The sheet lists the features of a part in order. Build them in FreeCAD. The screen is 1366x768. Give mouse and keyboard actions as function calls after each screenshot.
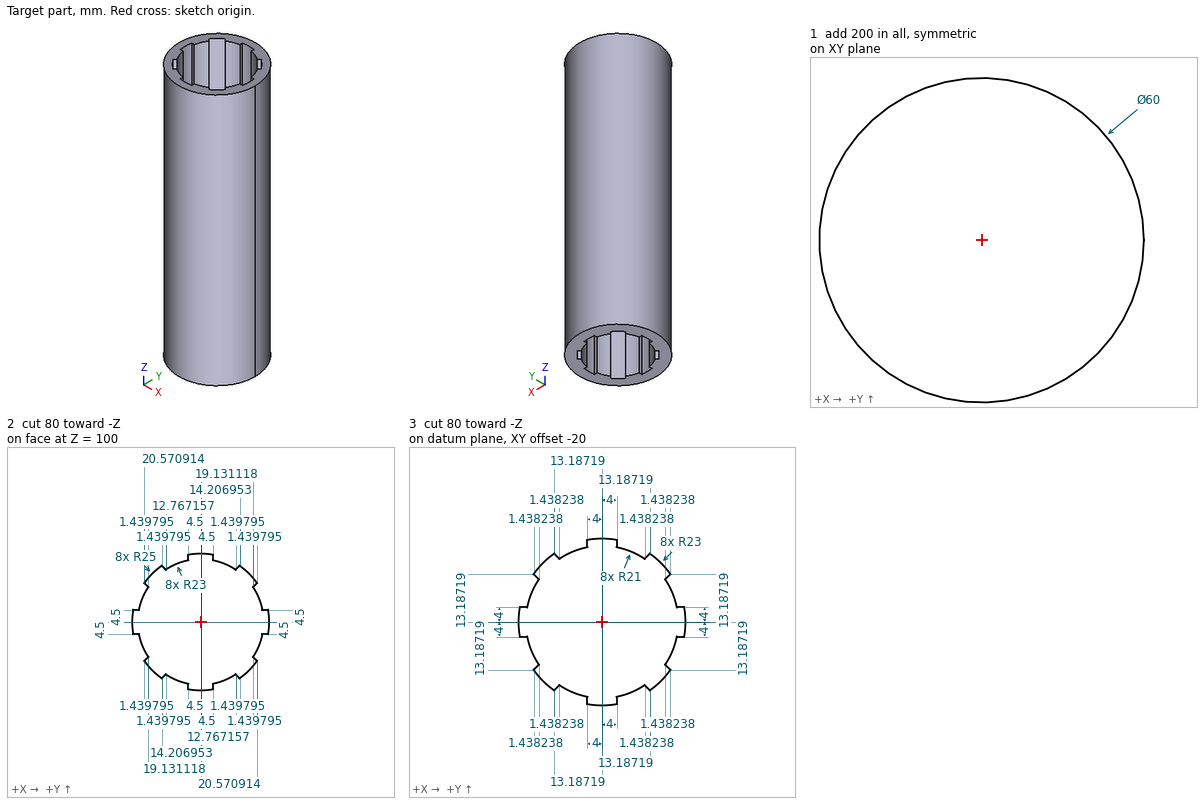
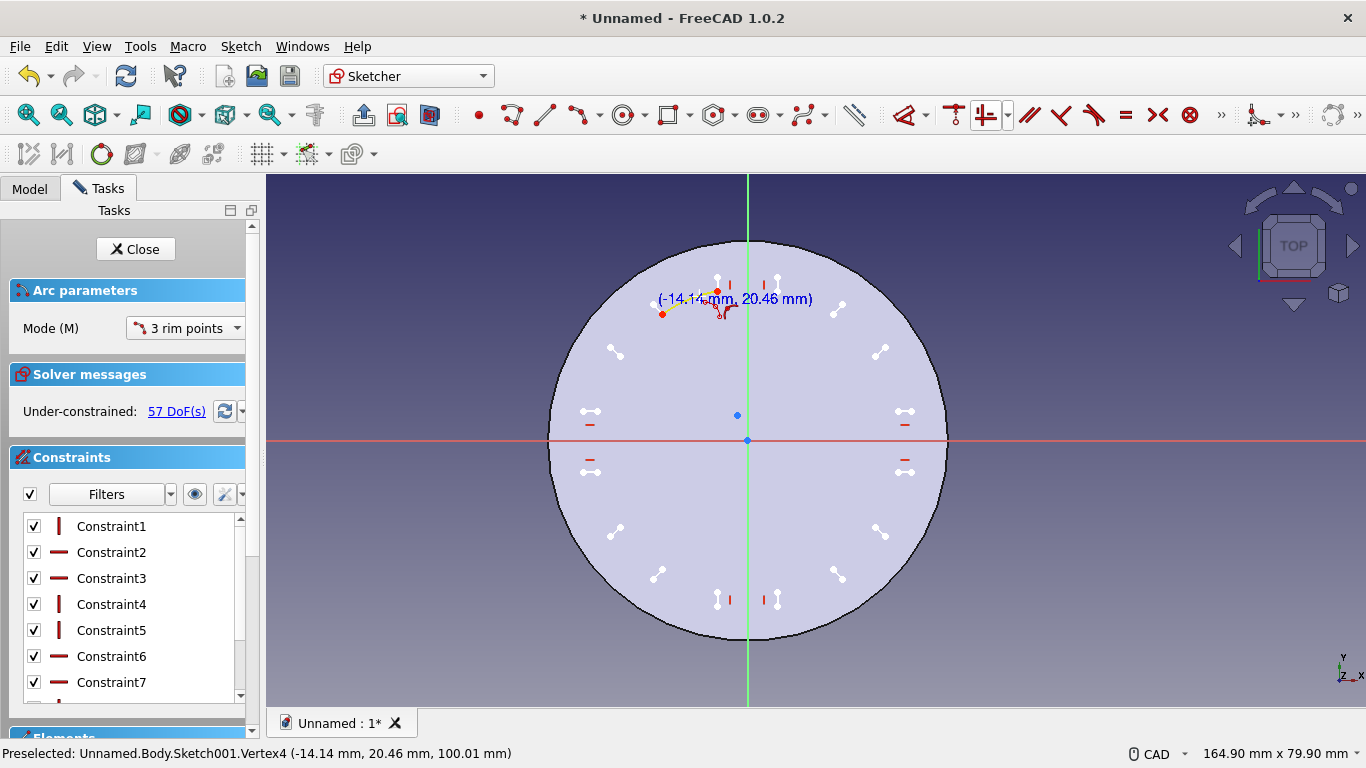
scroll(611, 346, up, 5)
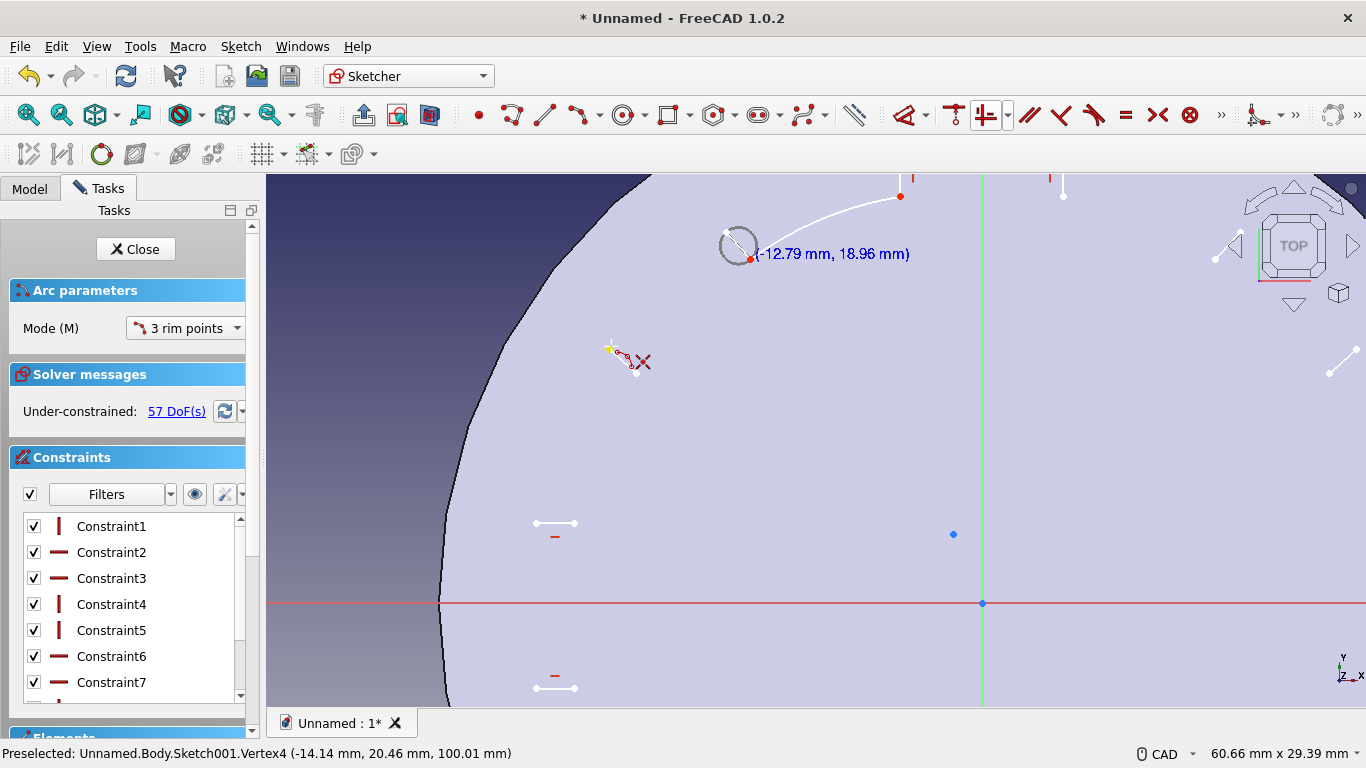
click(609, 349)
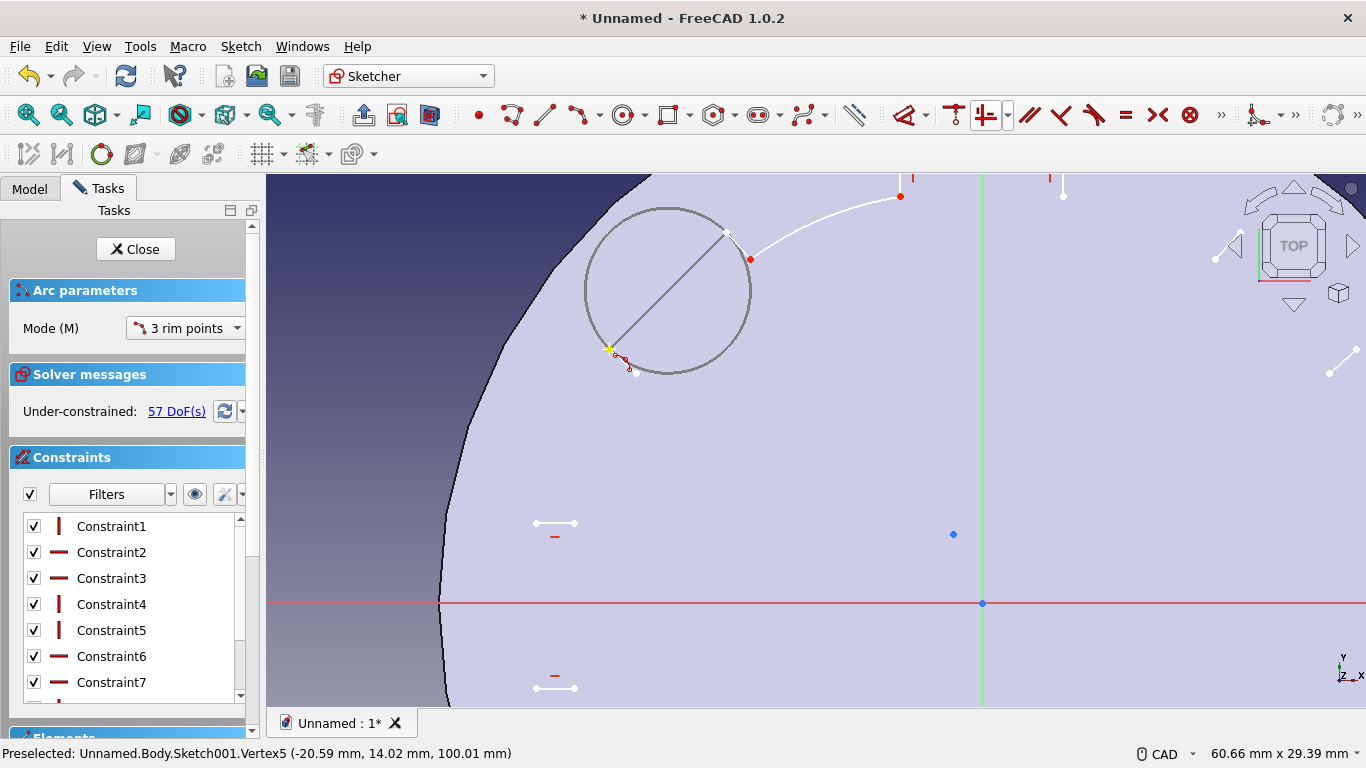
scroll(662, 283, up, 4)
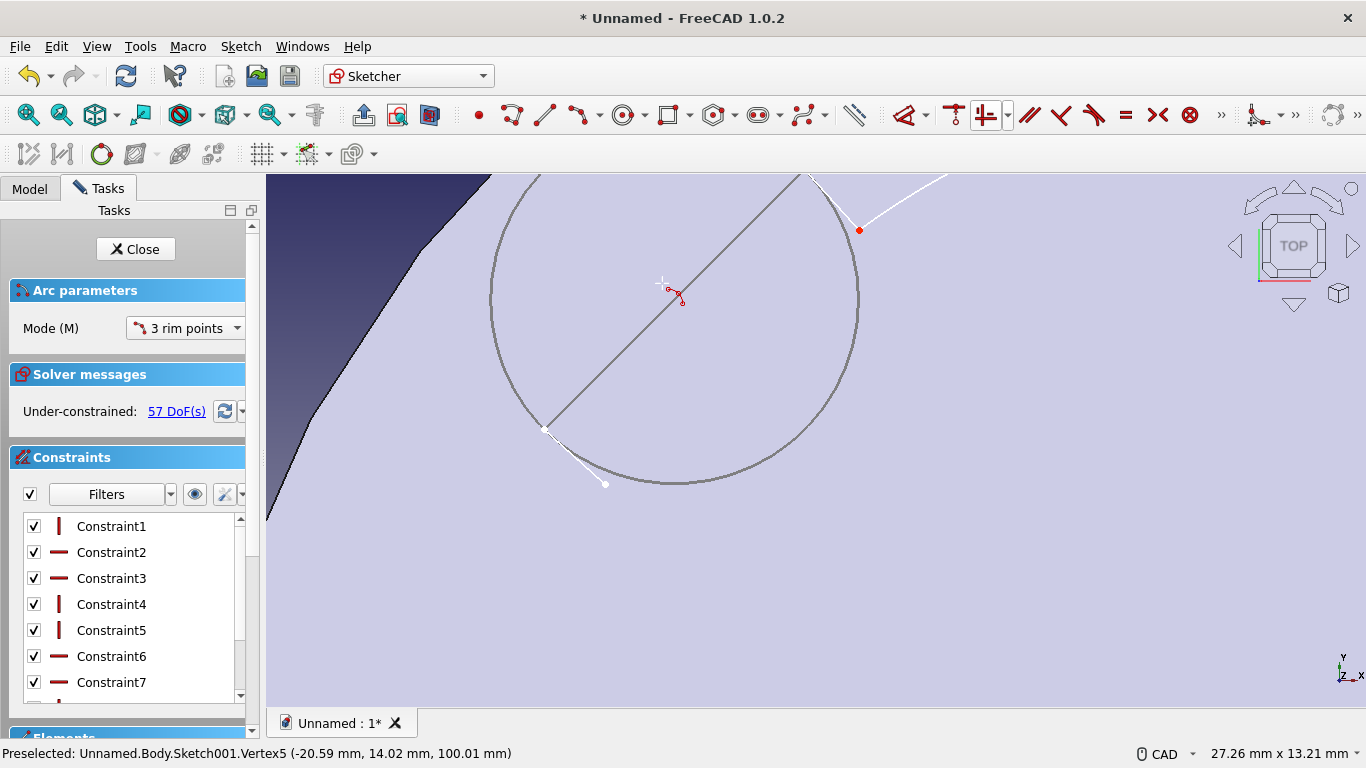
click(662, 282)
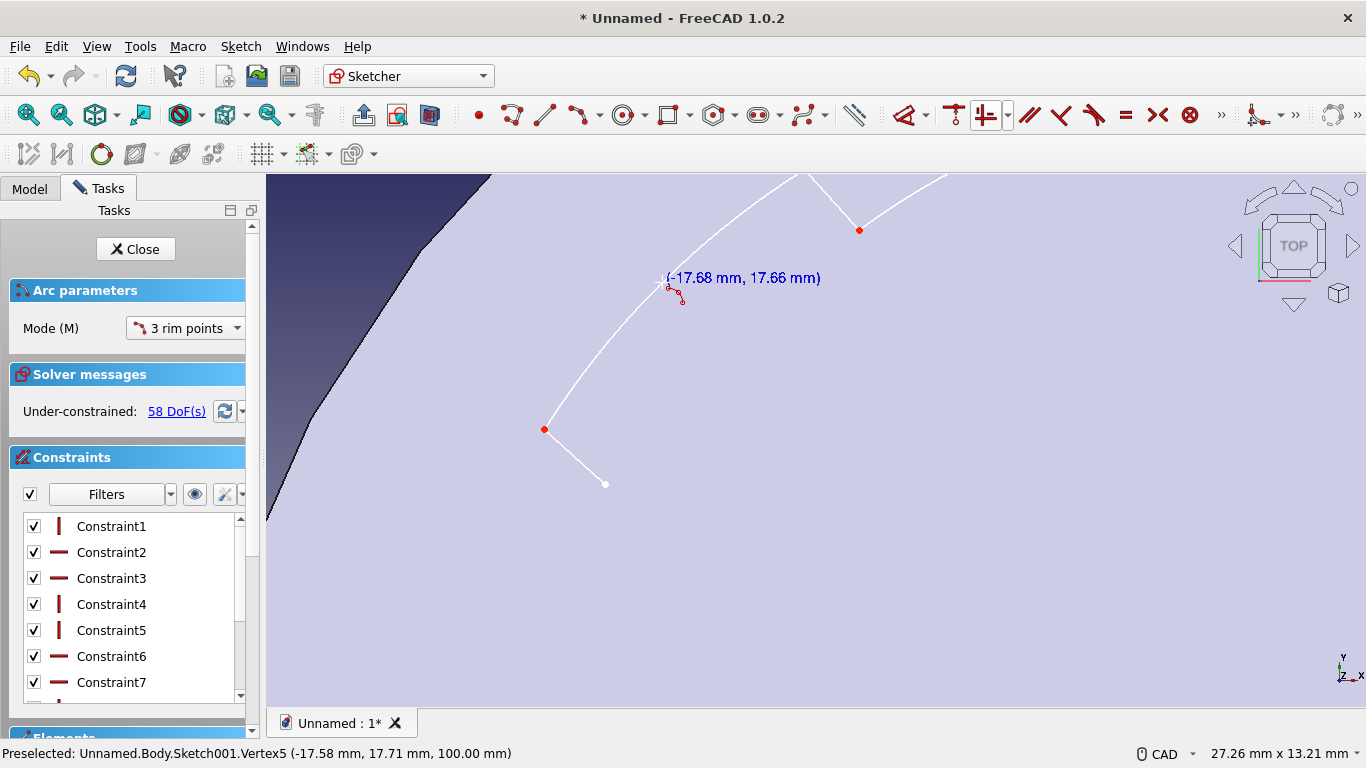
click(605, 484)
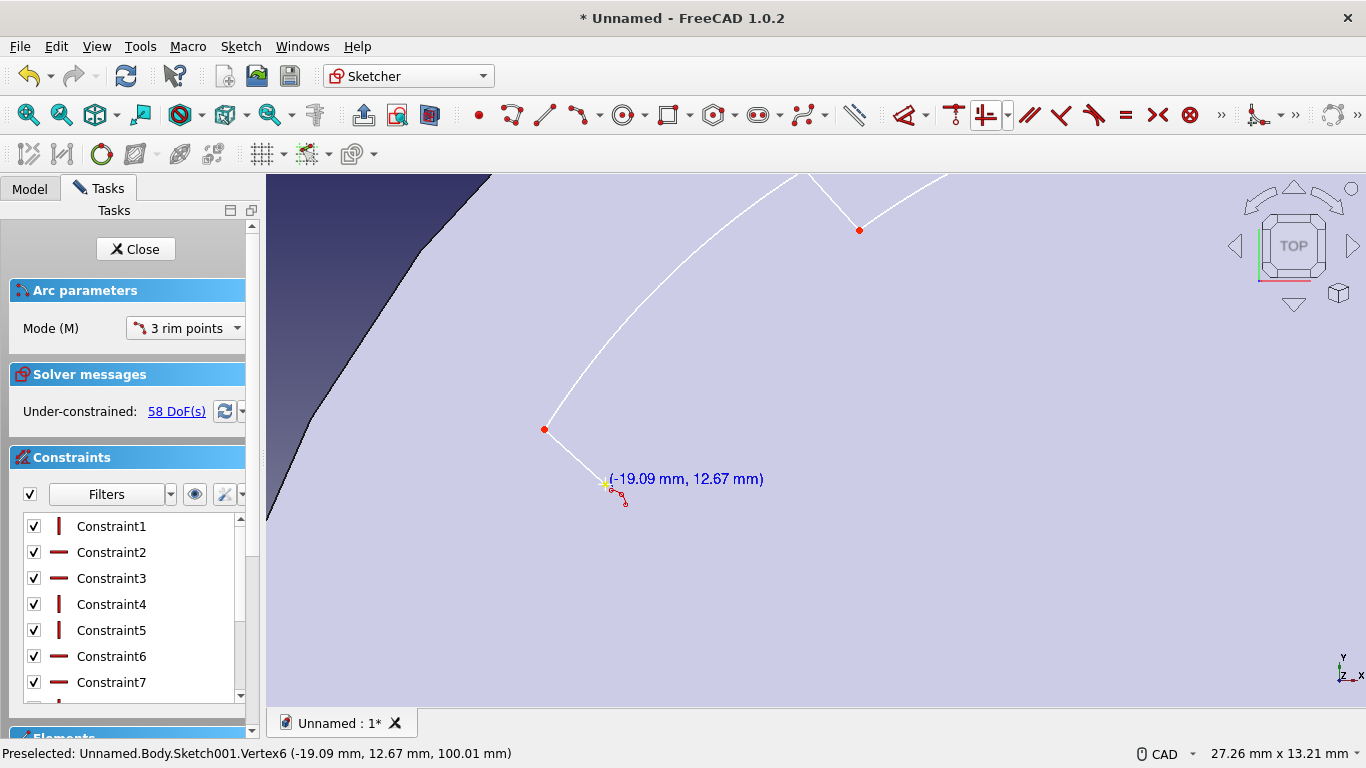
scroll(623, 331, down, 9)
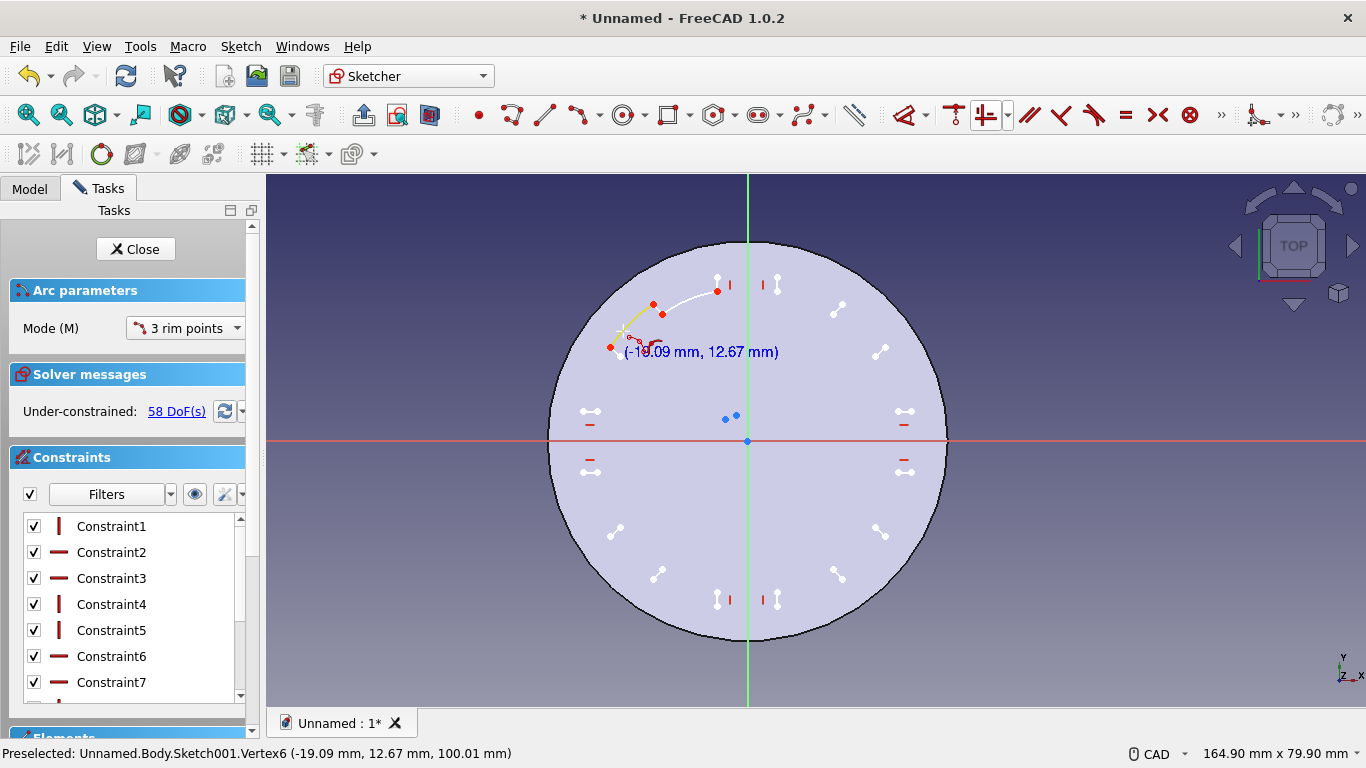
scroll(597, 411, up, 5)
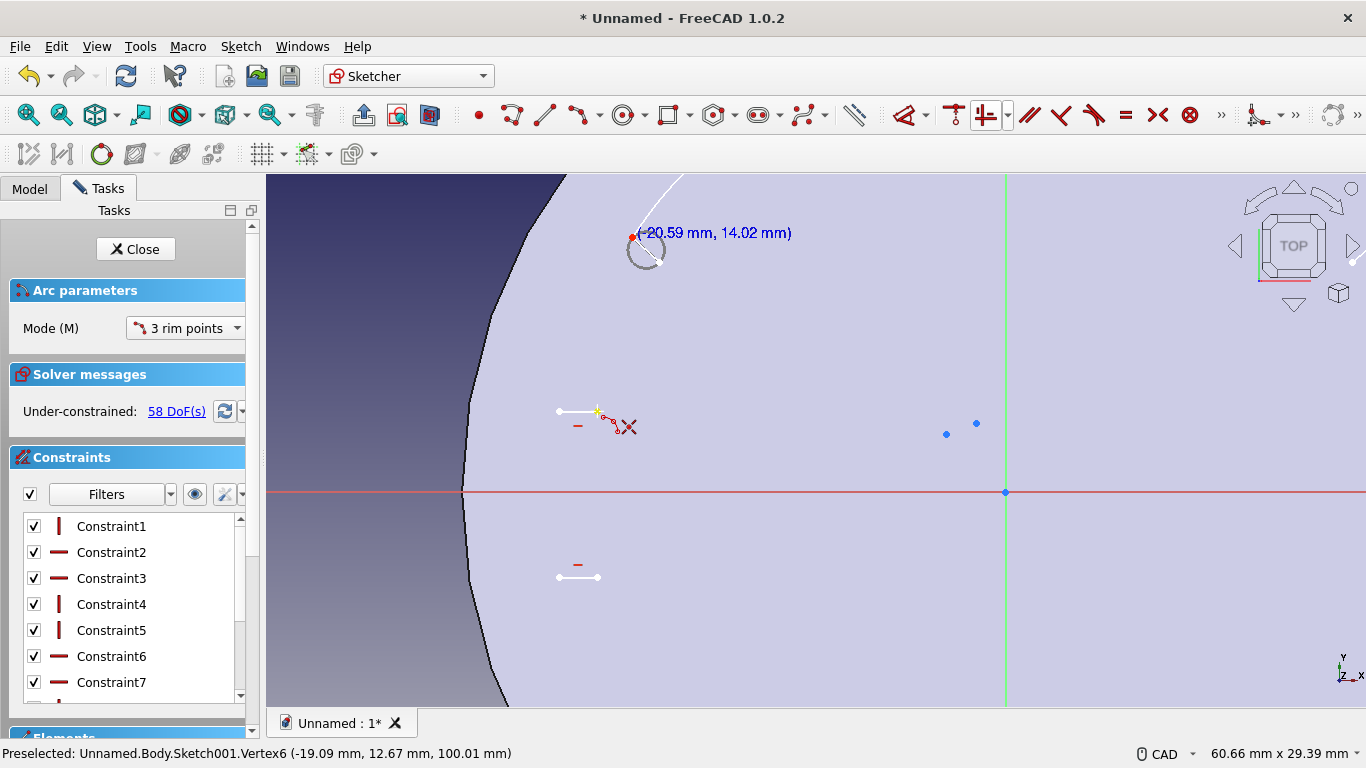
click(597, 412)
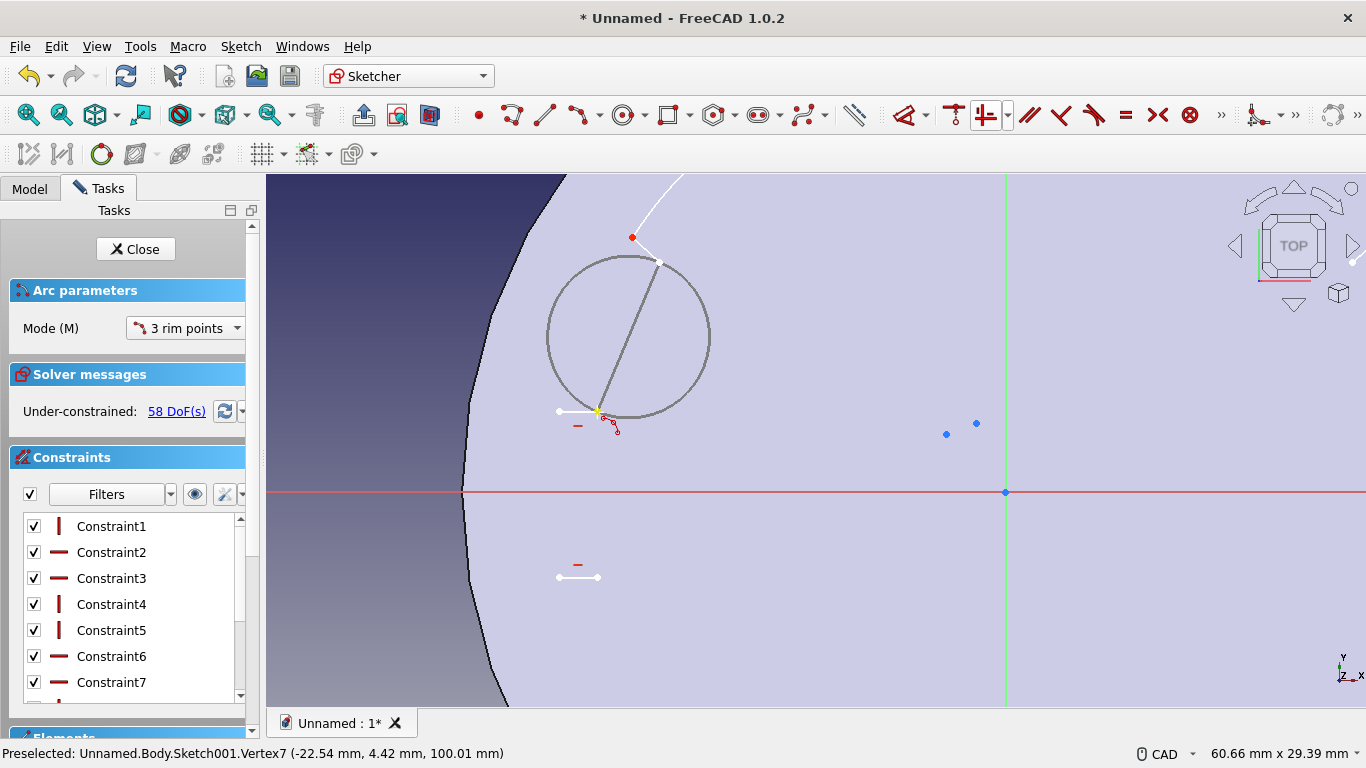
scroll(621, 332, up, 4)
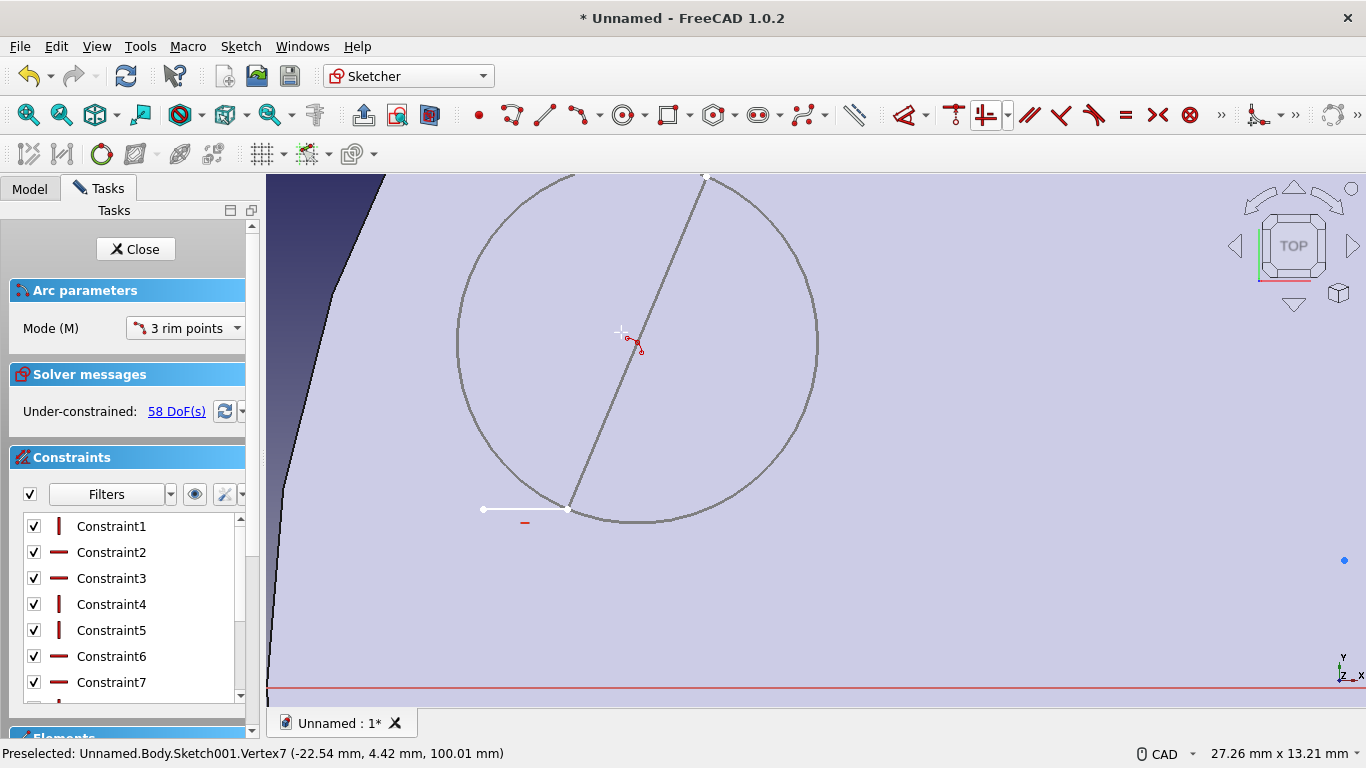
click(620, 333)